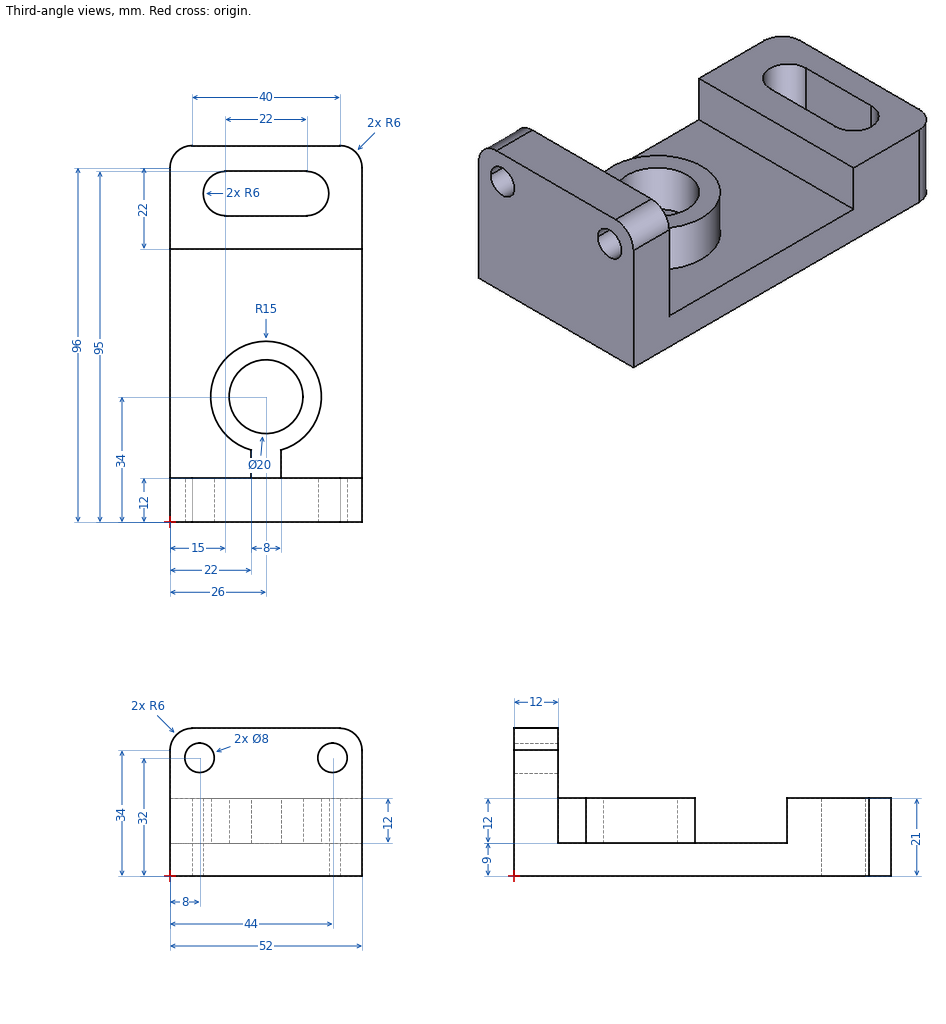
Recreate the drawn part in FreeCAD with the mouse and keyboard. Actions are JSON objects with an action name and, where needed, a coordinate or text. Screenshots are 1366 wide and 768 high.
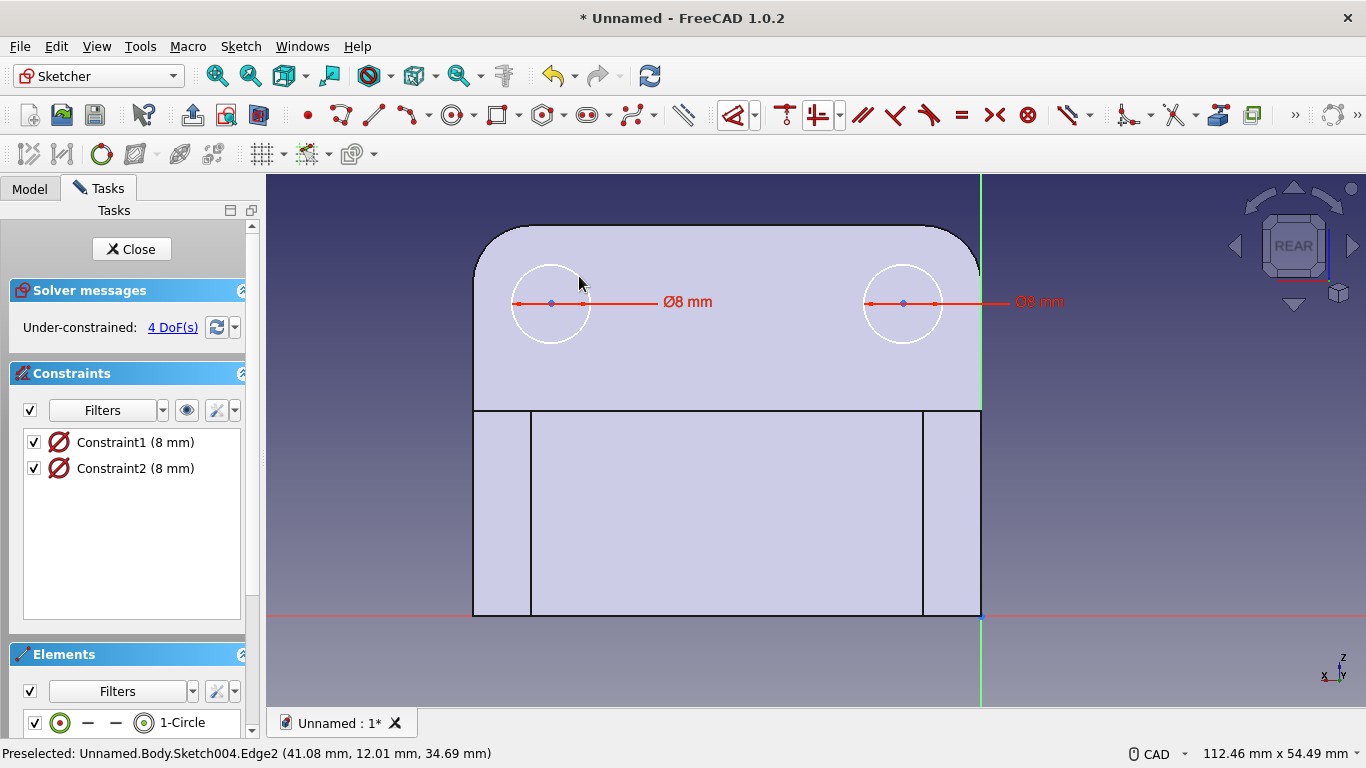
{"action": "left_click", "coordinate": [903, 304]}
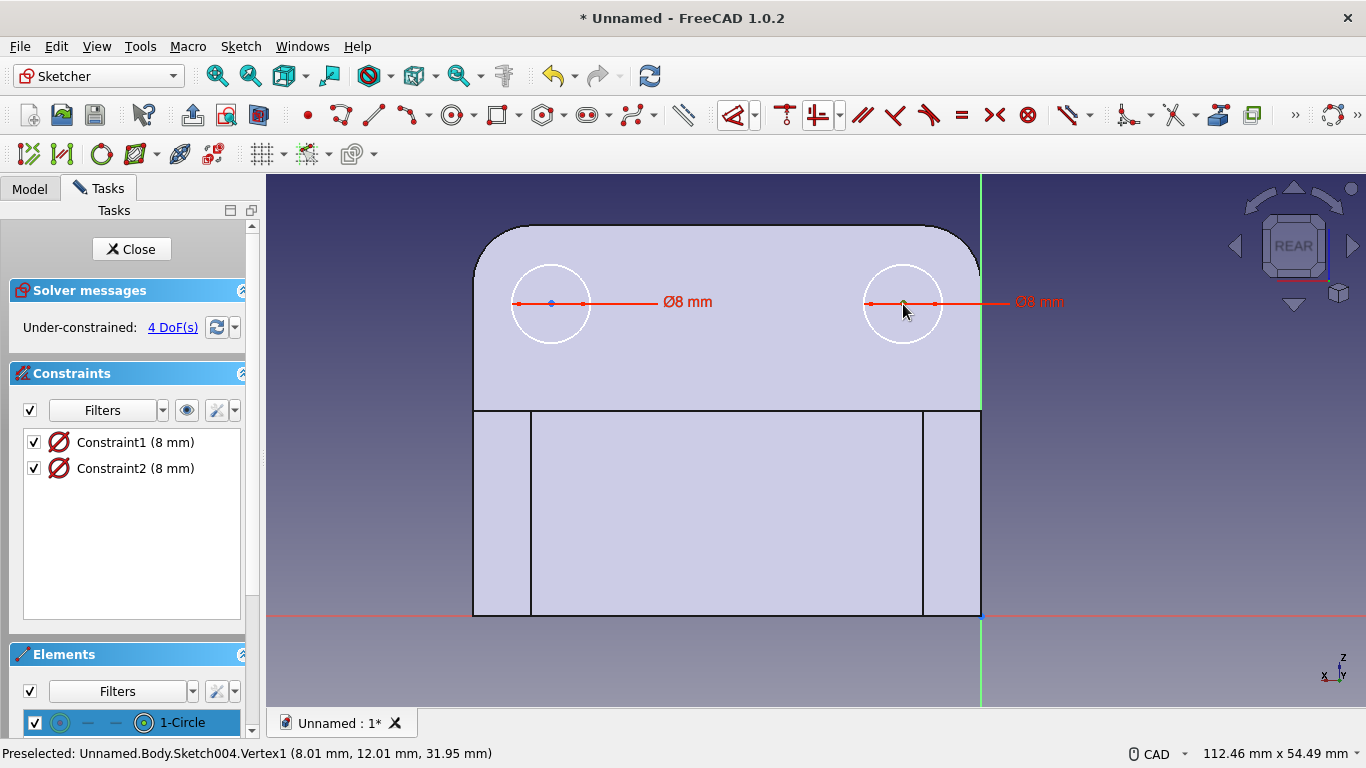
{"action": "left_click", "coordinate": [551, 304]}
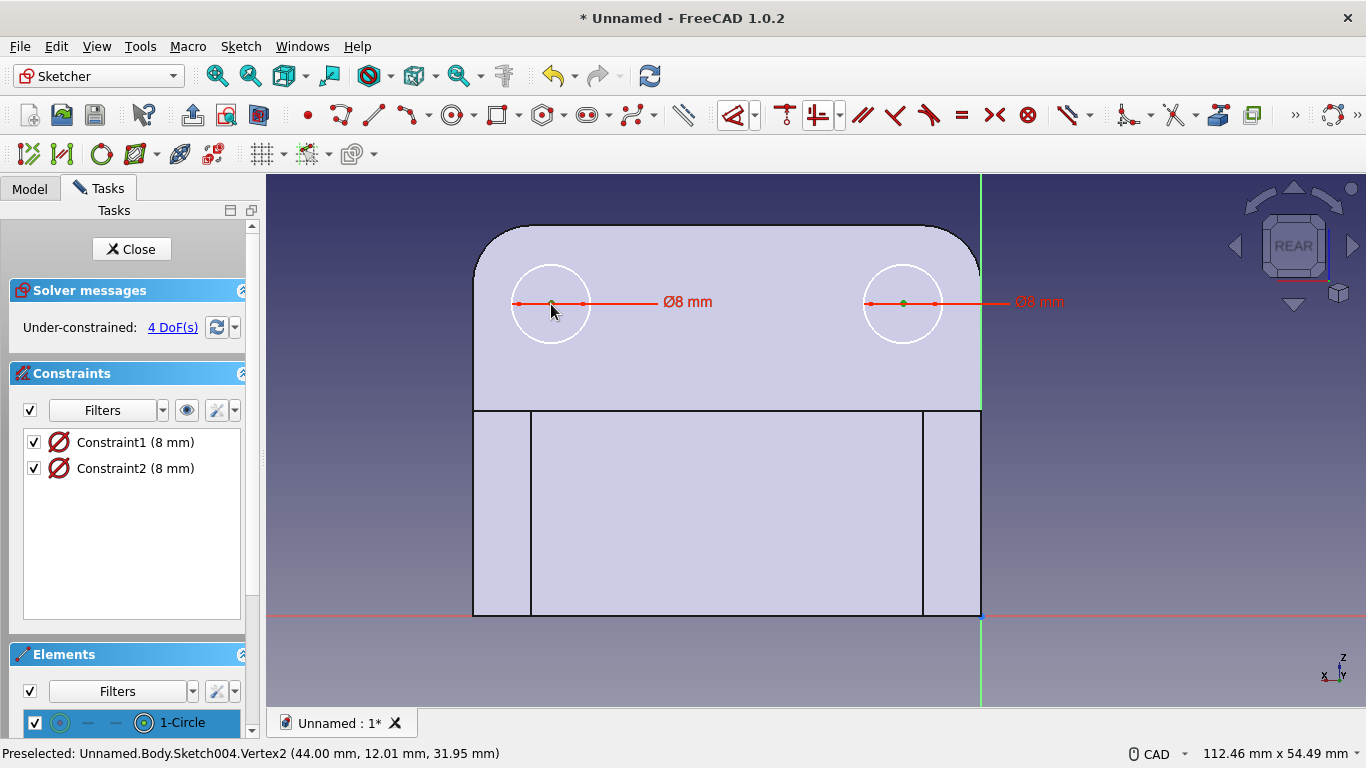
{"action": "key", "text": "h"}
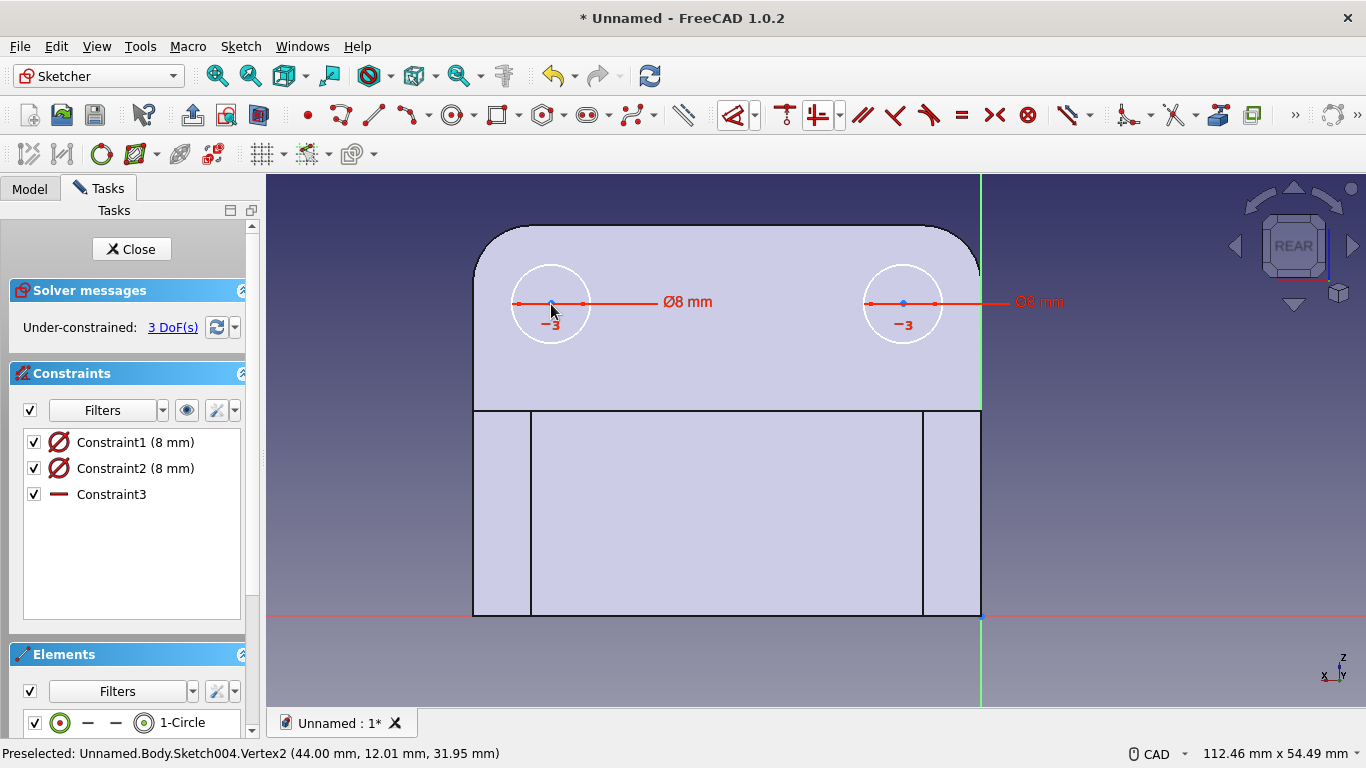
{"action": "left_click", "coordinate": [903, 304]}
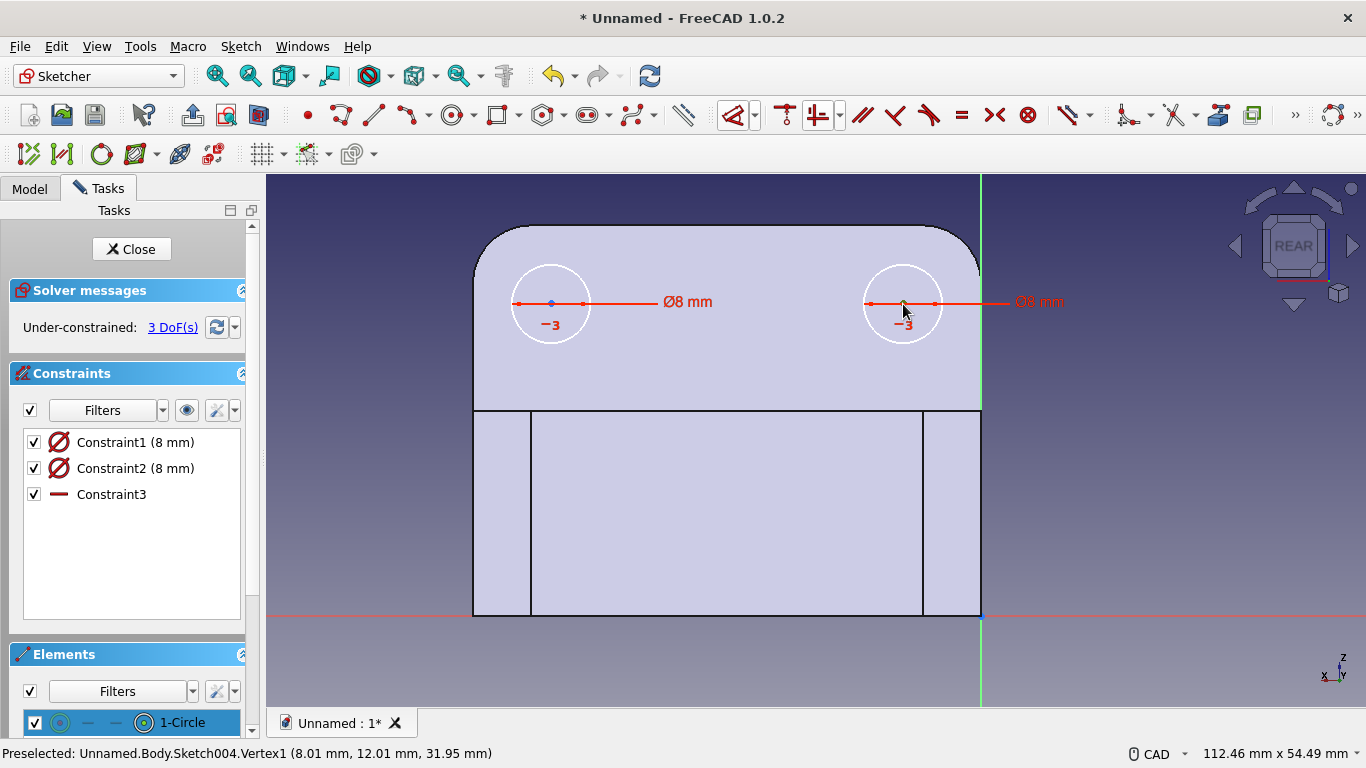
{"action": "key", "text": "l"}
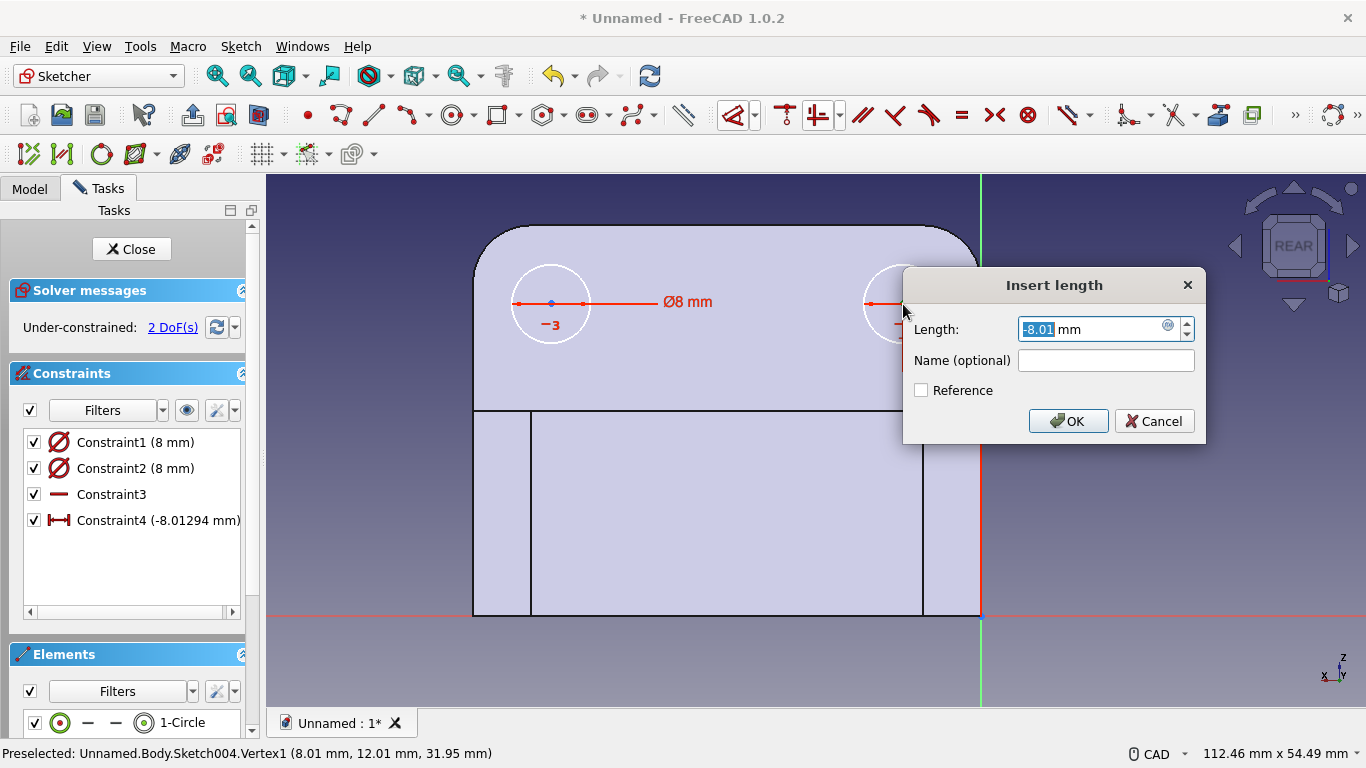
{"action": "type", "text": "-8"}
{"action": "key", "text": "Return"}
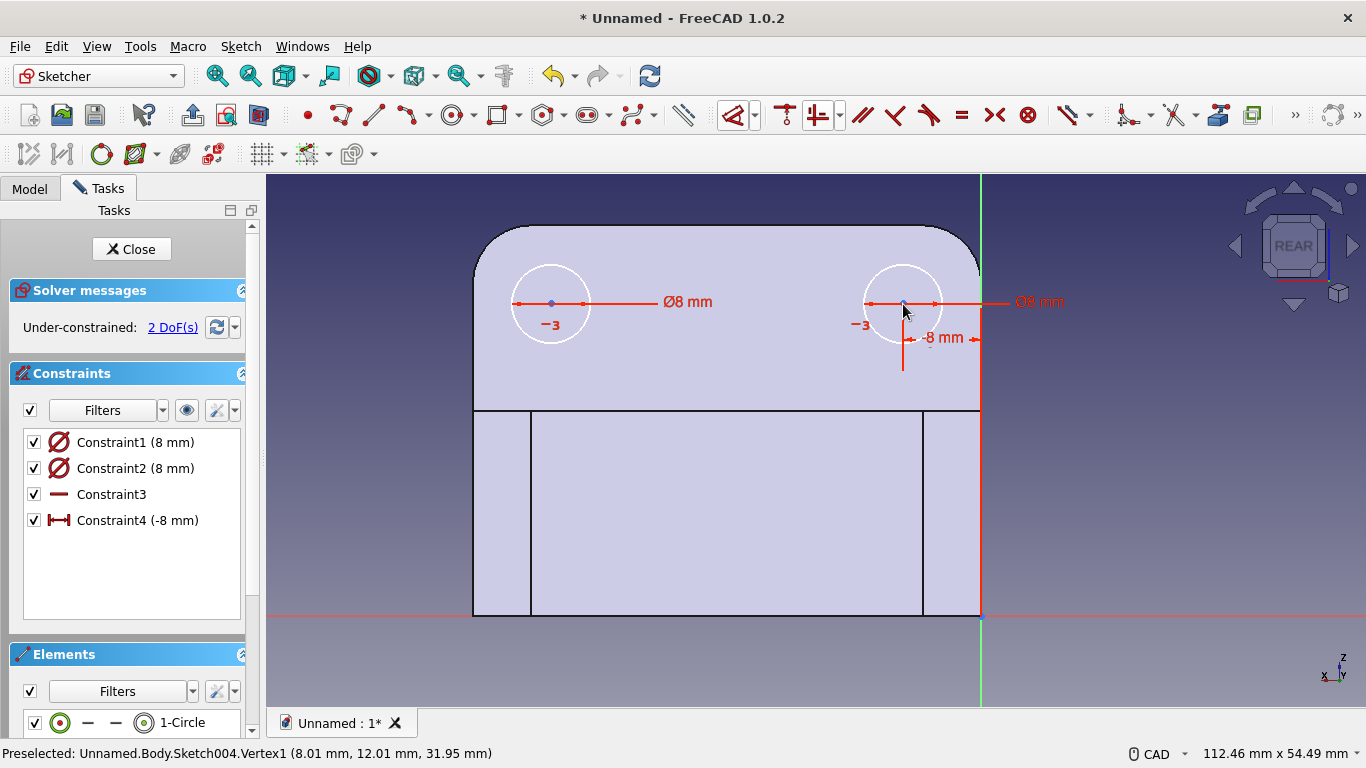
{"action": "left_click", "coordinate": [903, 304]}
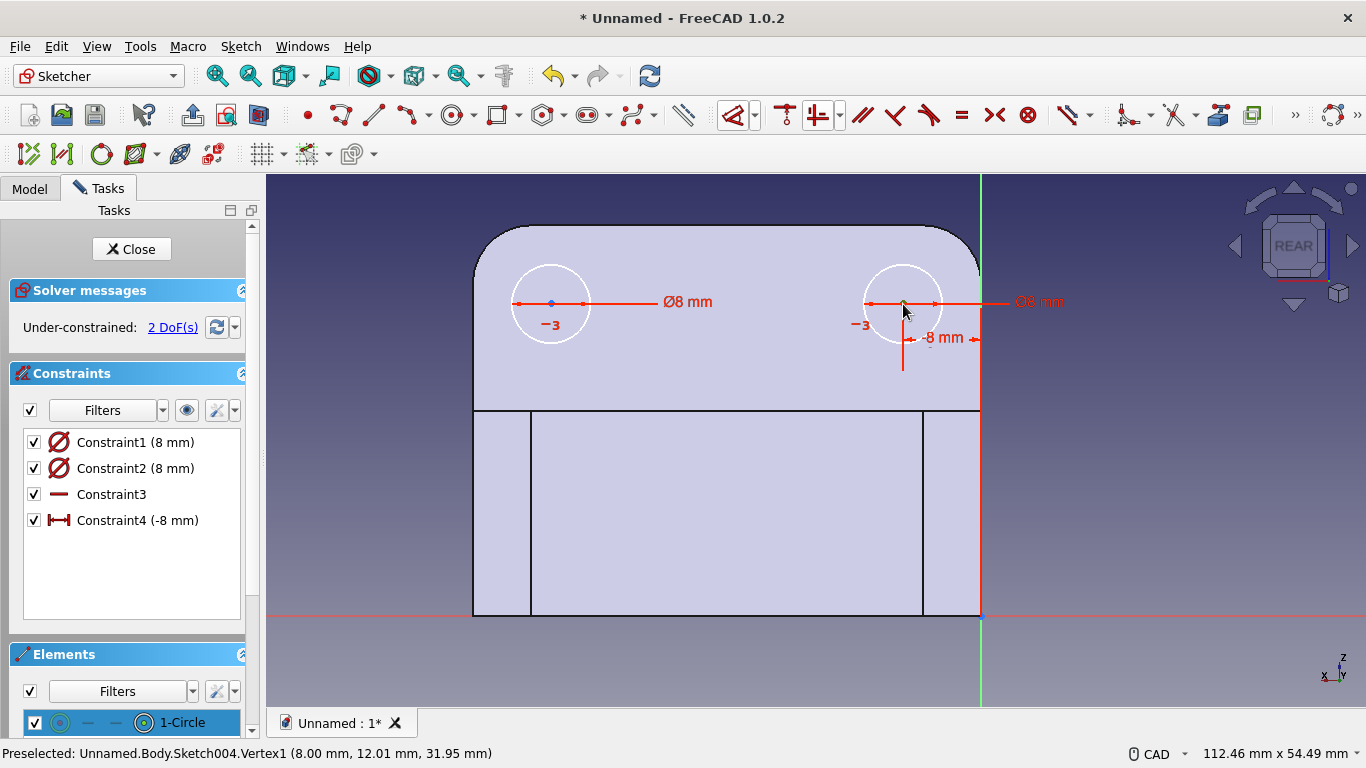
{"action": "left_click", "coordinate": [754, 116]}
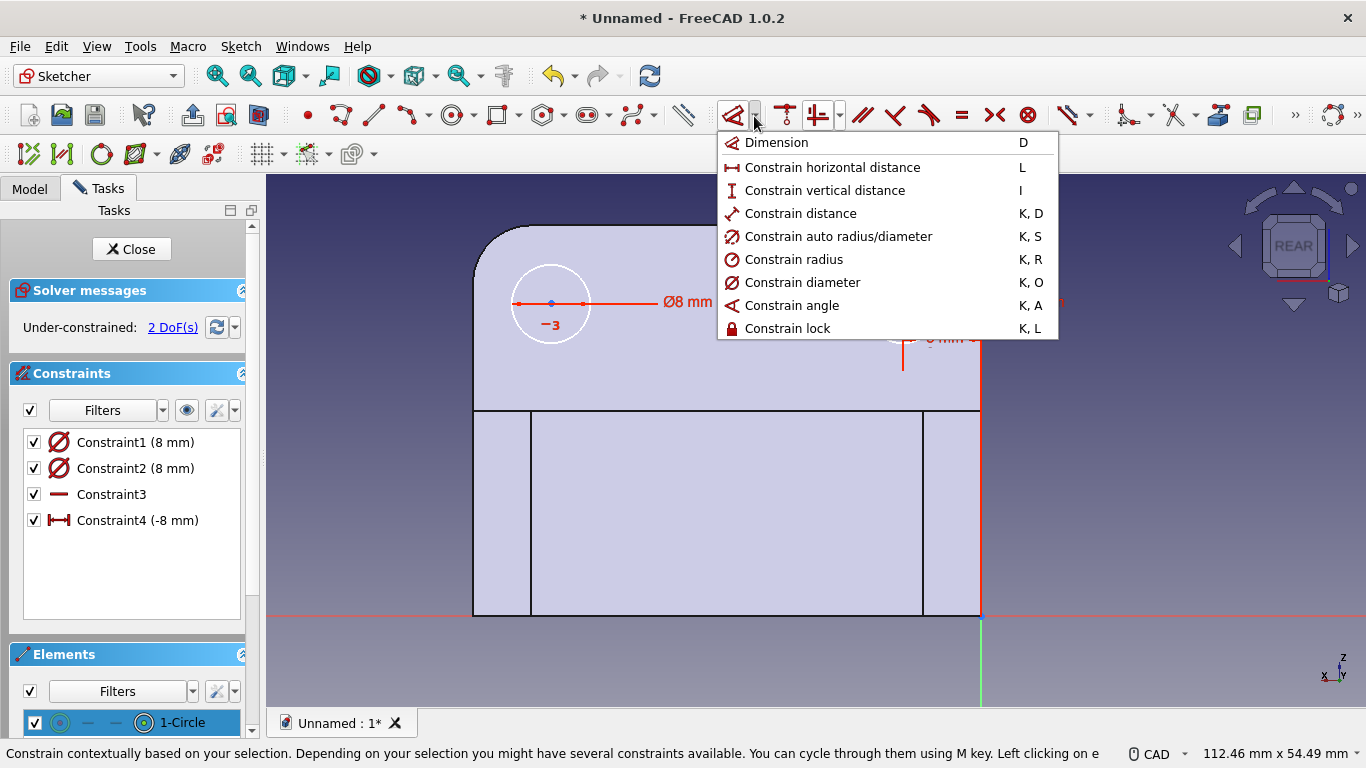
{"action": "left_click", "coordinate": [888, 190]}